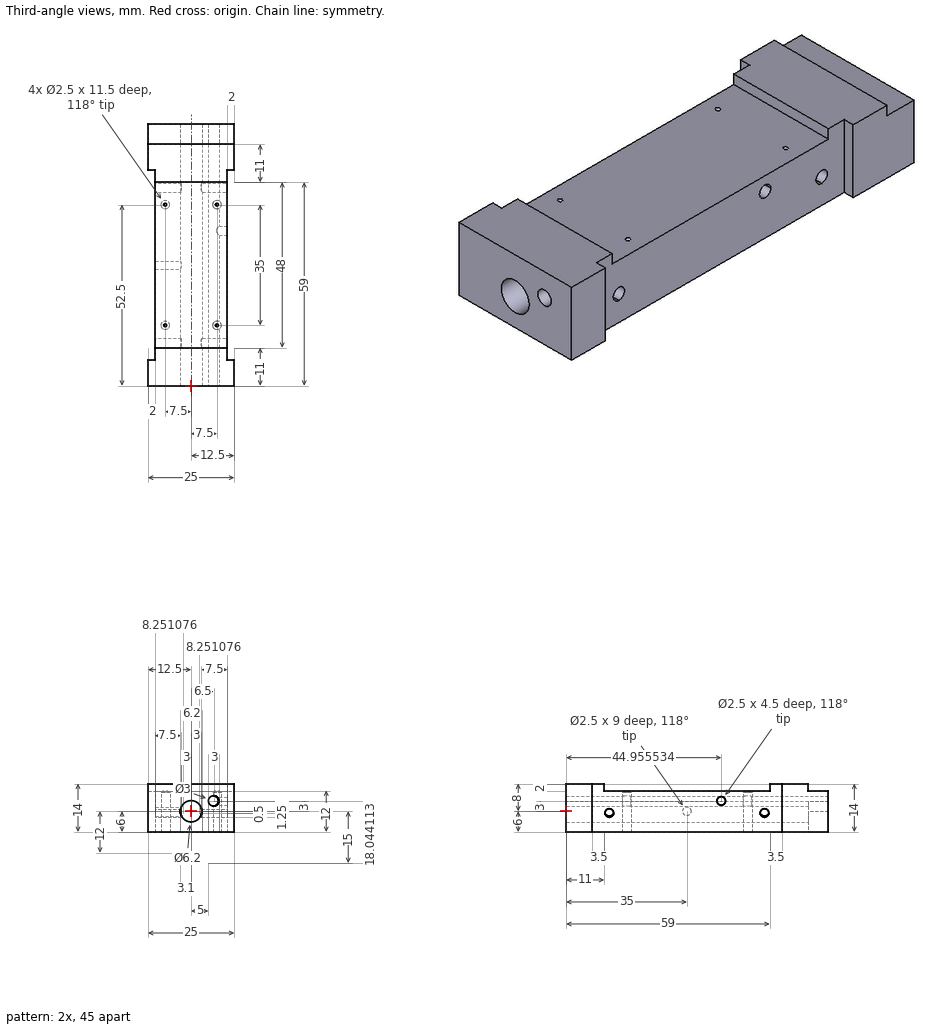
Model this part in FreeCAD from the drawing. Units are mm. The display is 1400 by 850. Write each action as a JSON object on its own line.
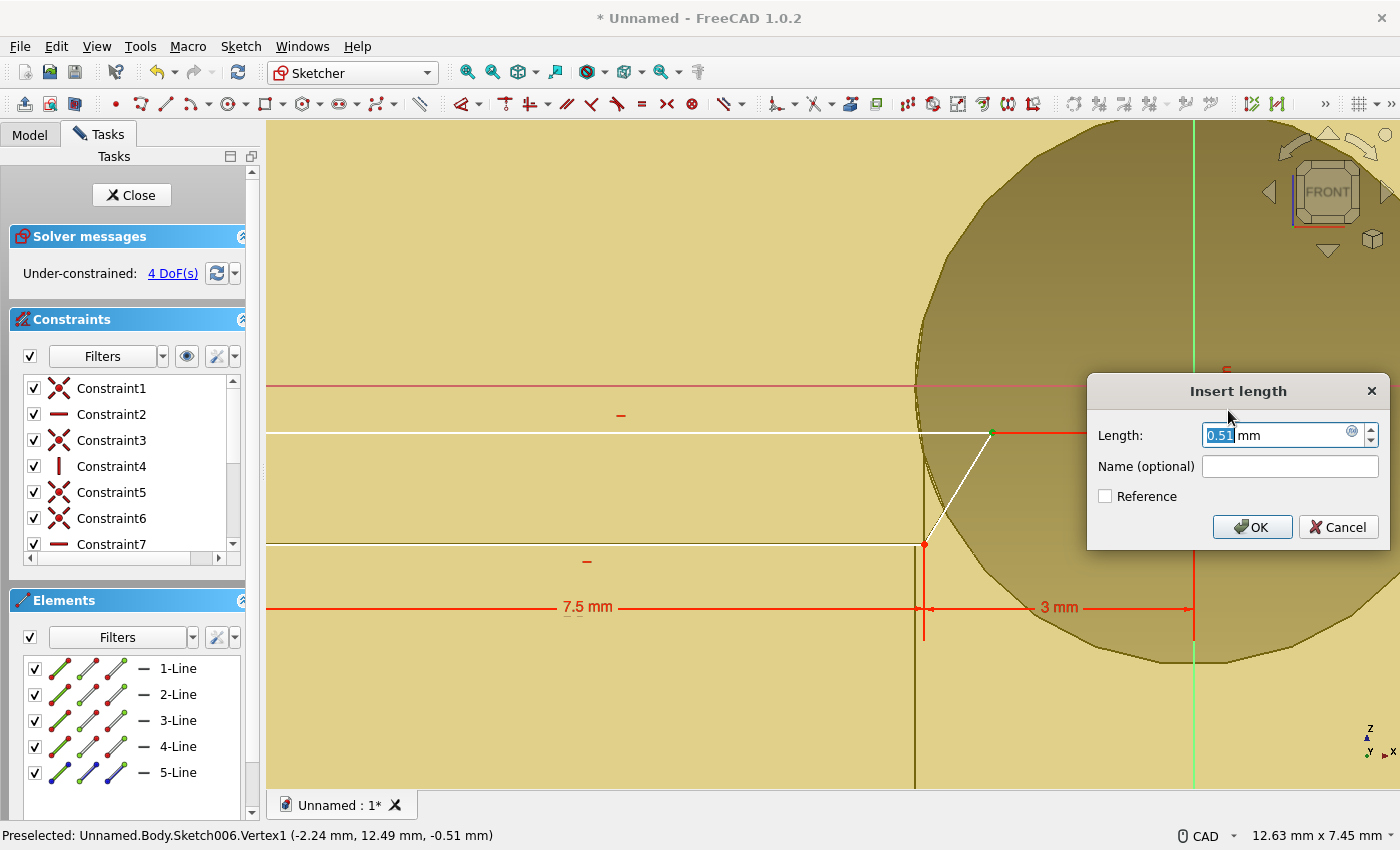
{"action": "type", "text": "0.5"}
{"action": "key", "text": "Return"}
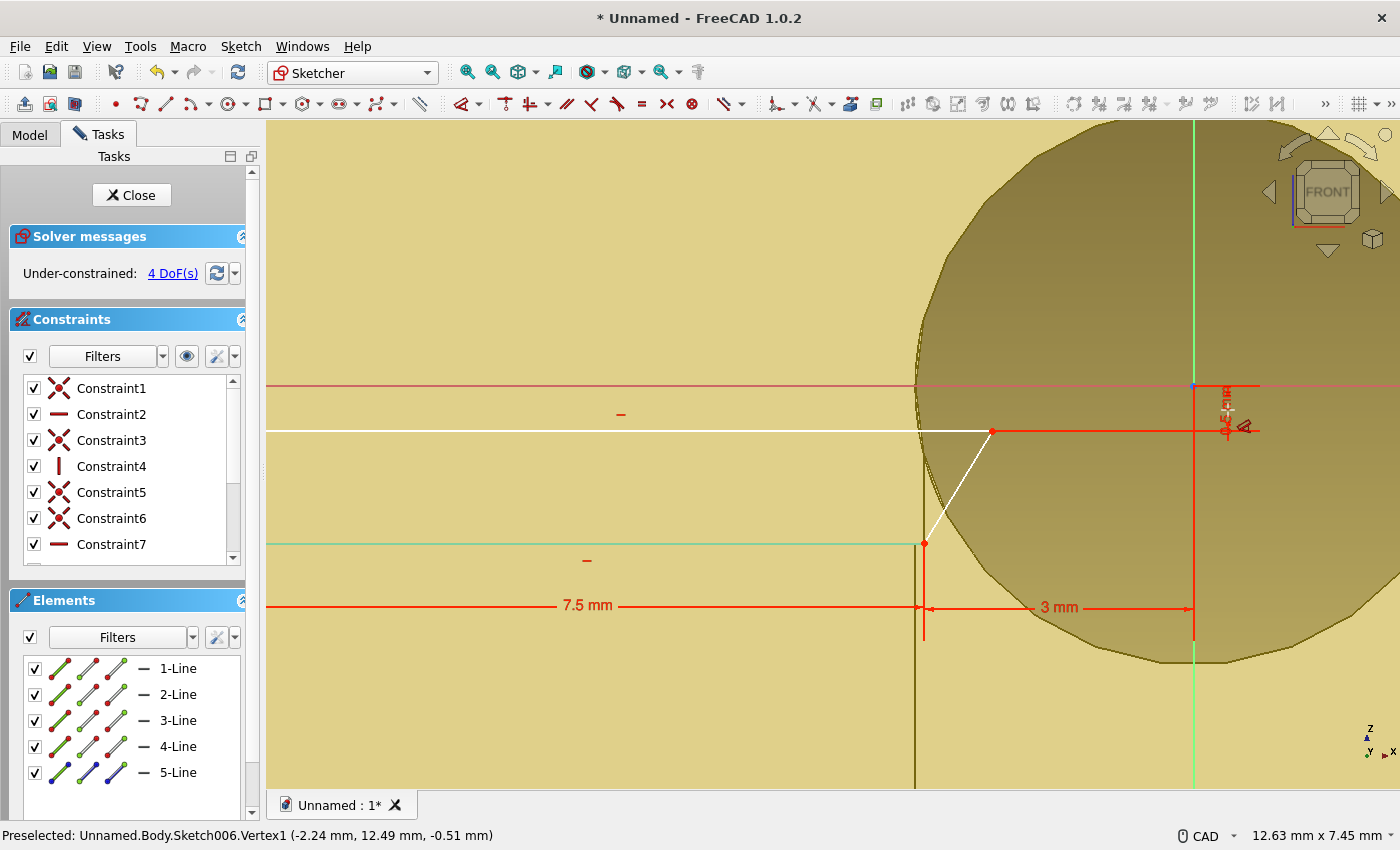
{"action": "scroll", "coordinate": [996, 442], "scroll_direction": "down", "scroll_amount": 3}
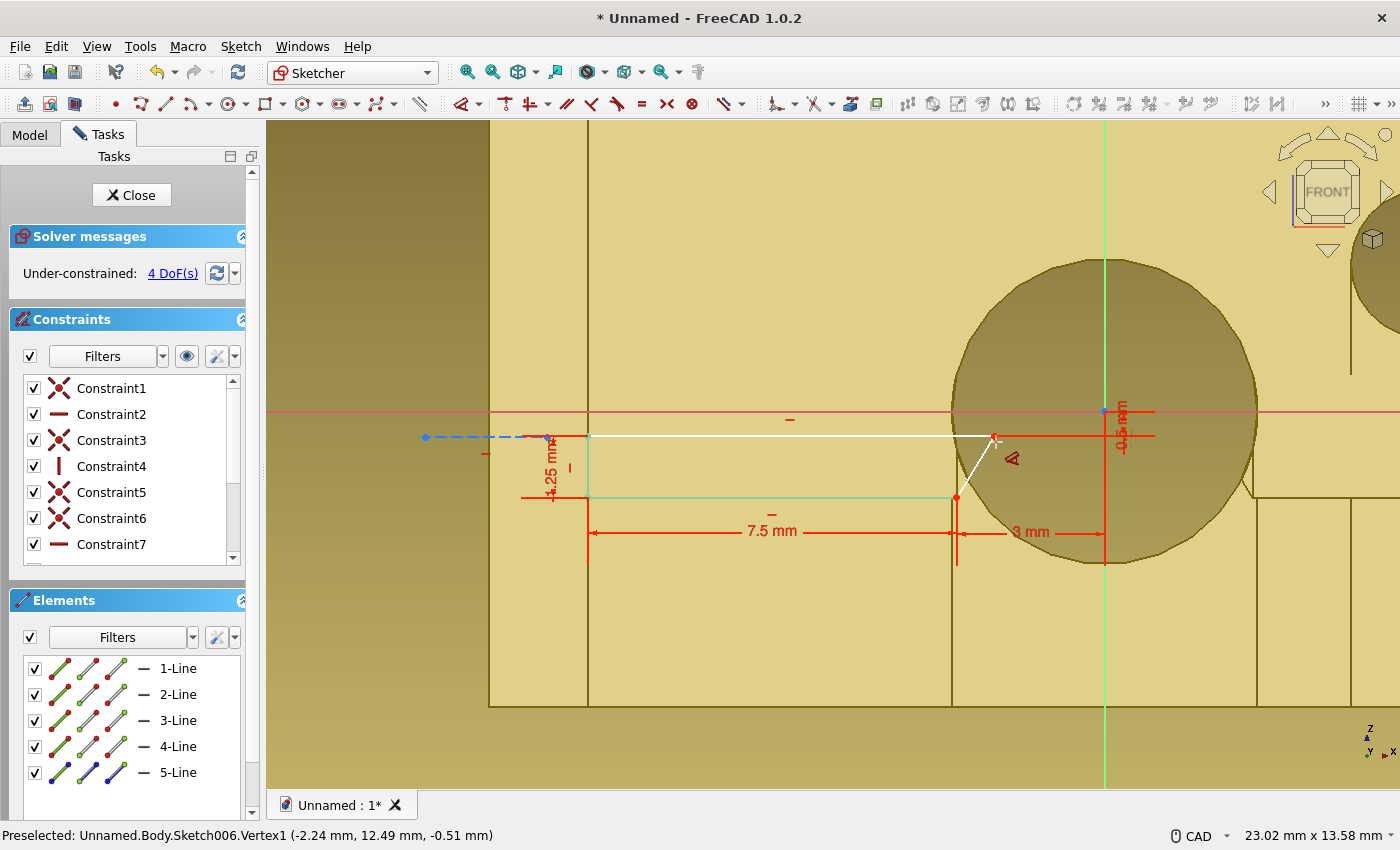
{"action": "scroll", "coordinate": [547, 437], "scroll_direction": "up", "scroll_amount": 3}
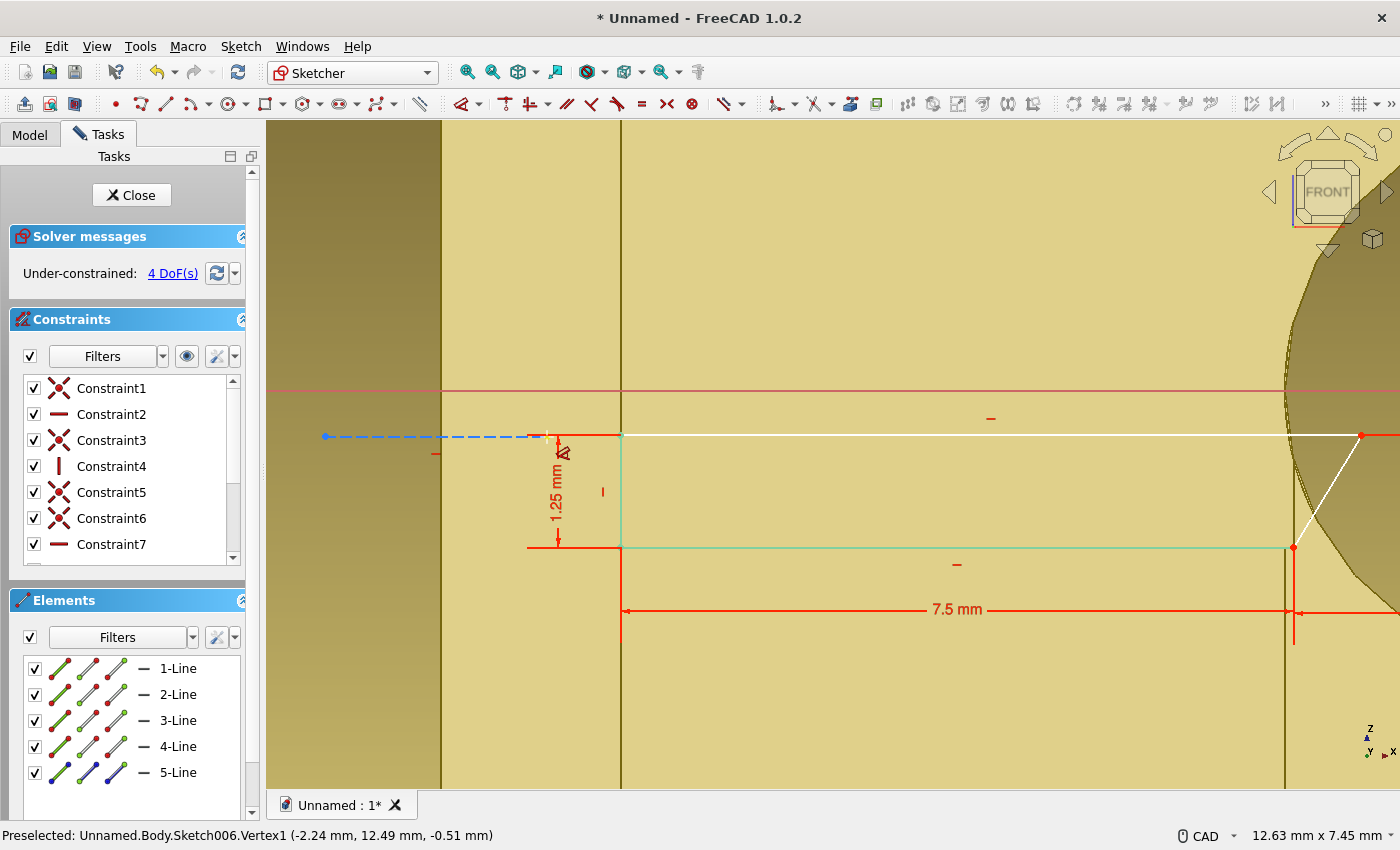
{"action": "left_click", "coordinate": [547, 437]}
{"action": "left_click", "coordinate": [513, 414]}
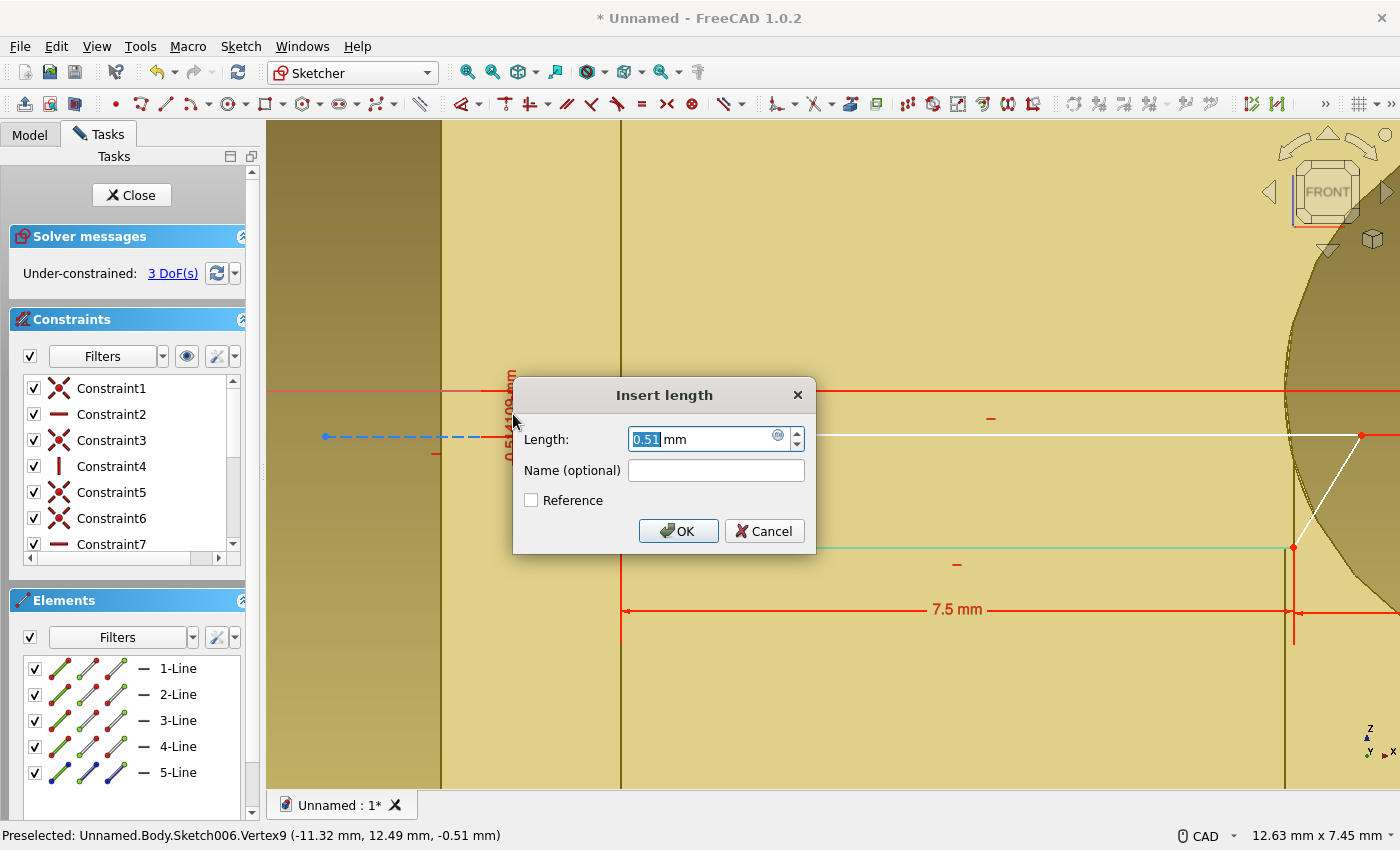
{"action": "type", "text": "0.5"}
{"action": "key", "text": "Return"}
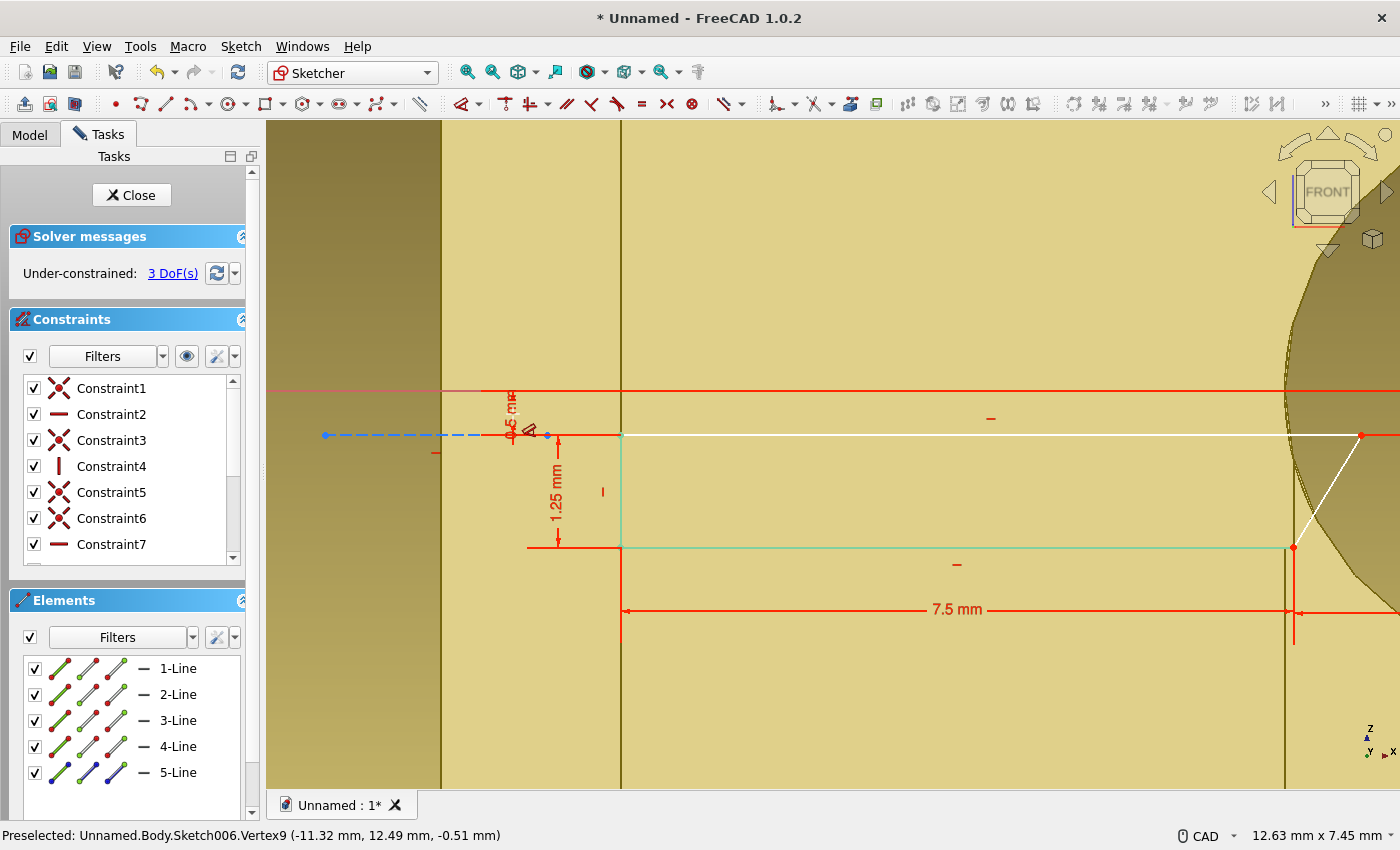
{"action": "left_click", "coordinate": [843, 435]}
{"action": "left_click", "coordinate": [928, 469]}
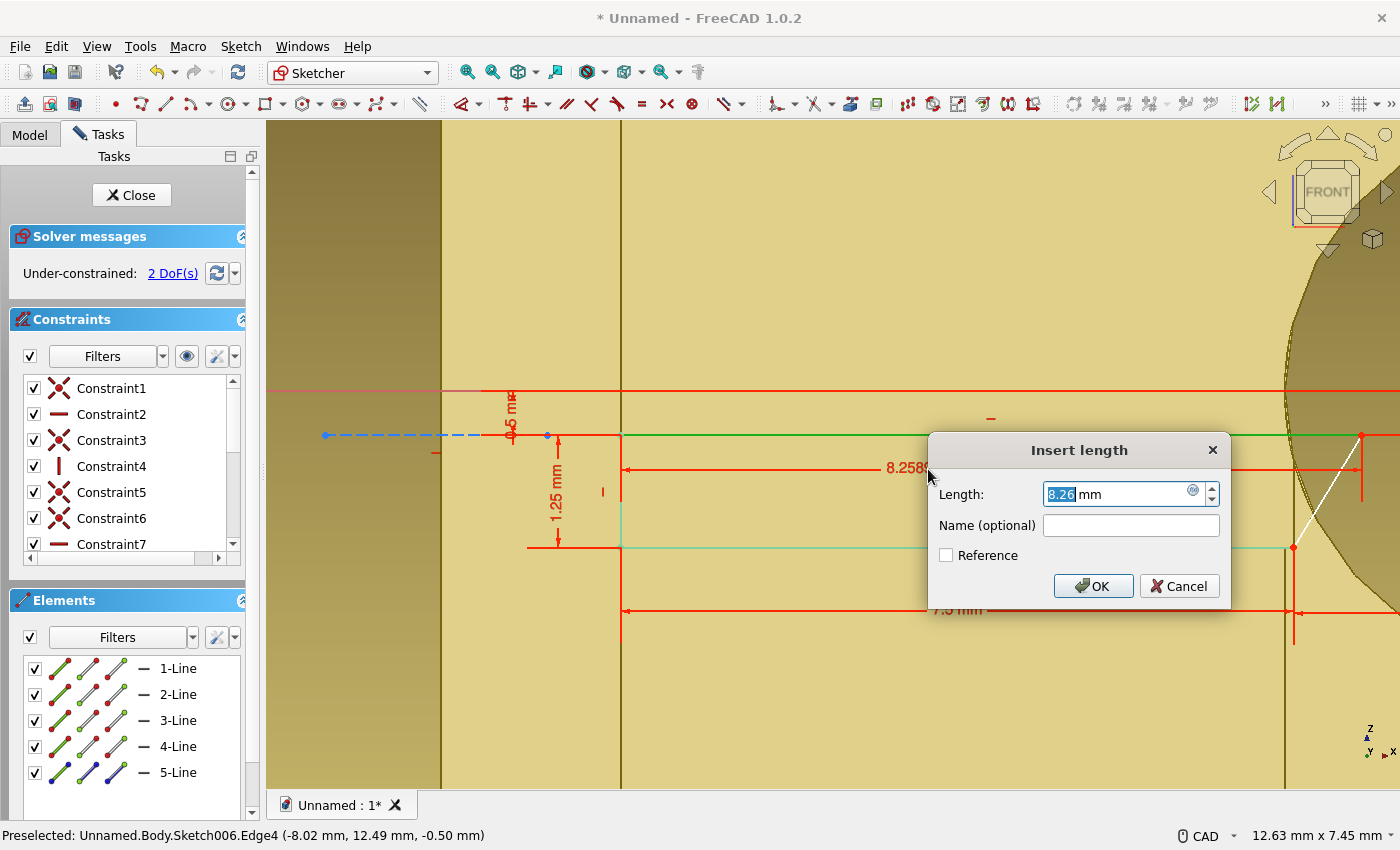
{"action": "type", "text": "8.251076"}
{"action": "key", "text": "Return"}
{"action": "key", "text": "Escape"}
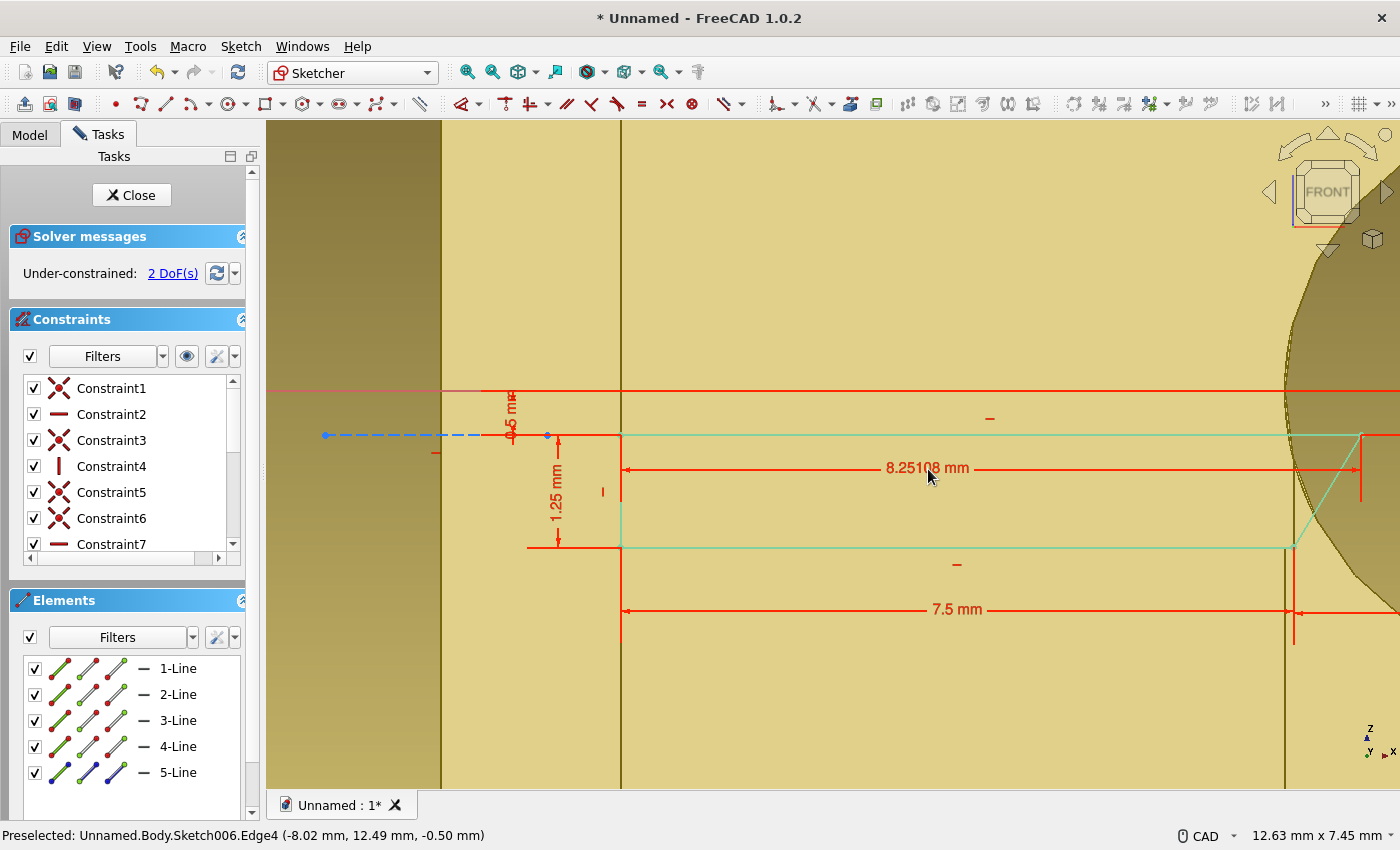
{"action": "left_click", "coordinate": [132, 195]}